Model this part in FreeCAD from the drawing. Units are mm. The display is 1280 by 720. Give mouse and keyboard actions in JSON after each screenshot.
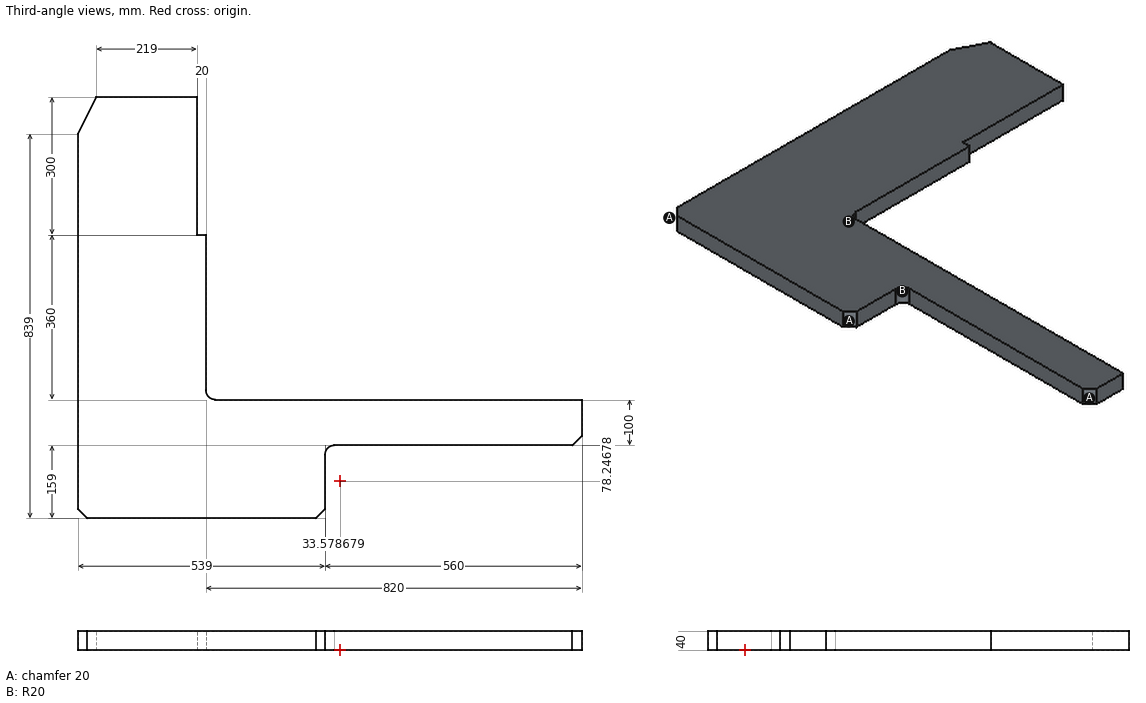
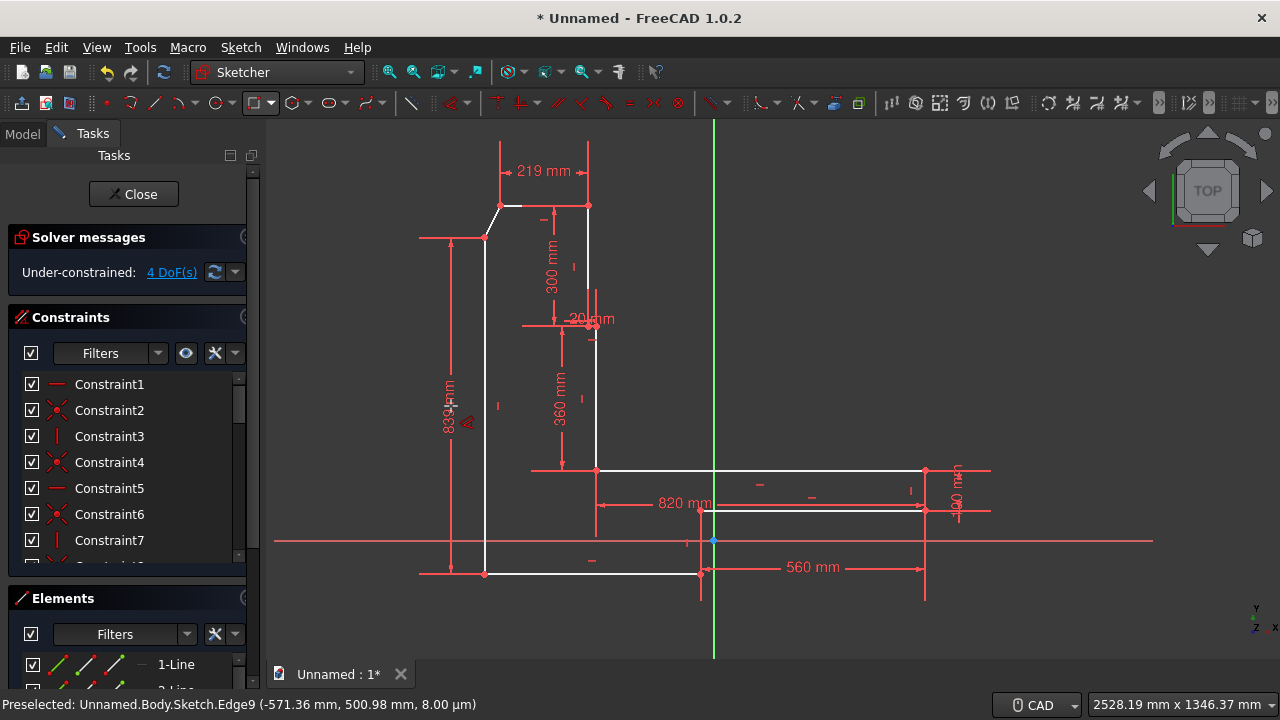
{"action": "left_click", "coordinate": [549, 574]}
{"action": "left_click", "coordinate": [593, 608]}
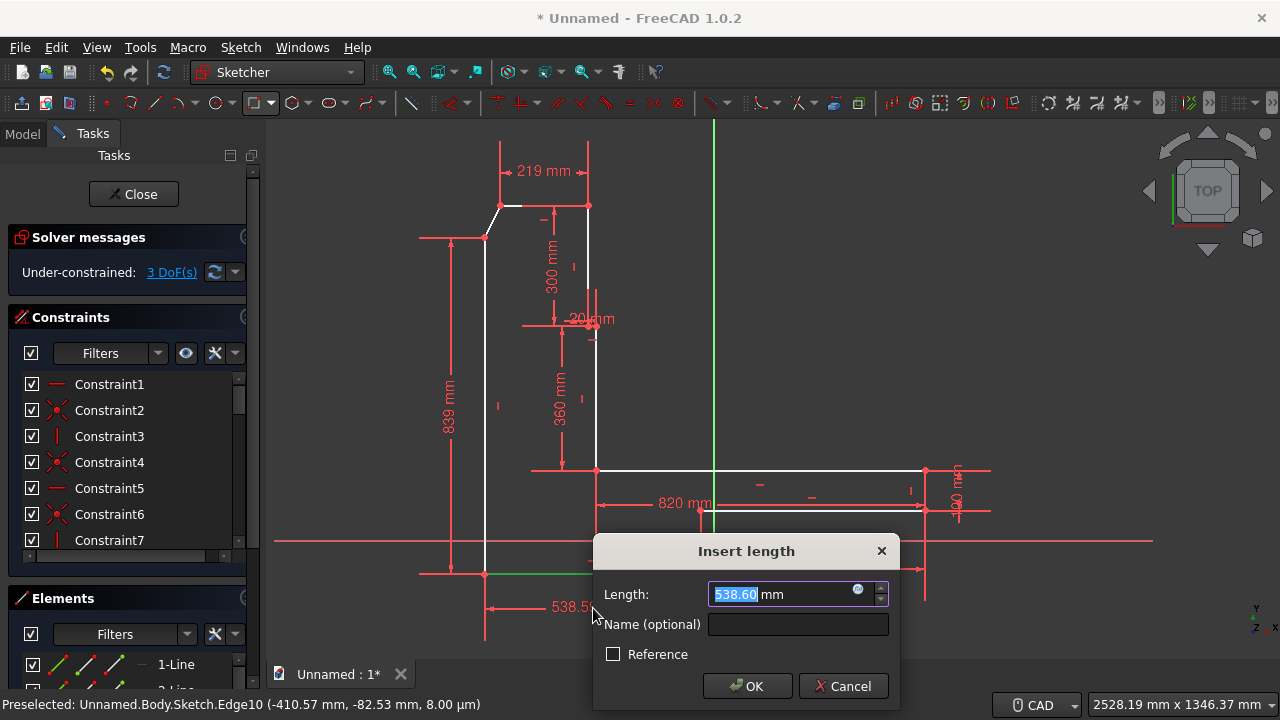
{"action": "type", "text": "539"}
{"action": "key", "text": "Return"}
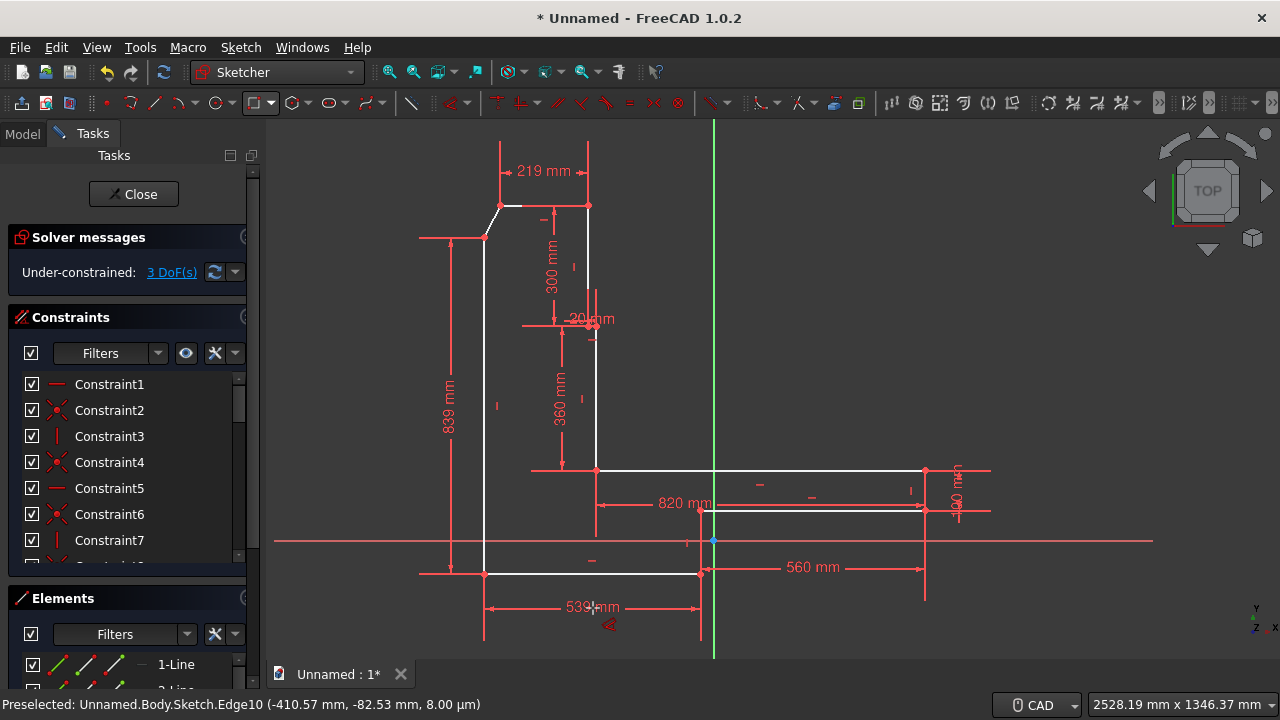
{"action": "left_click", "coordinate": [701, 555]}
{"action": "left_click", "coordinate": [667, 528]}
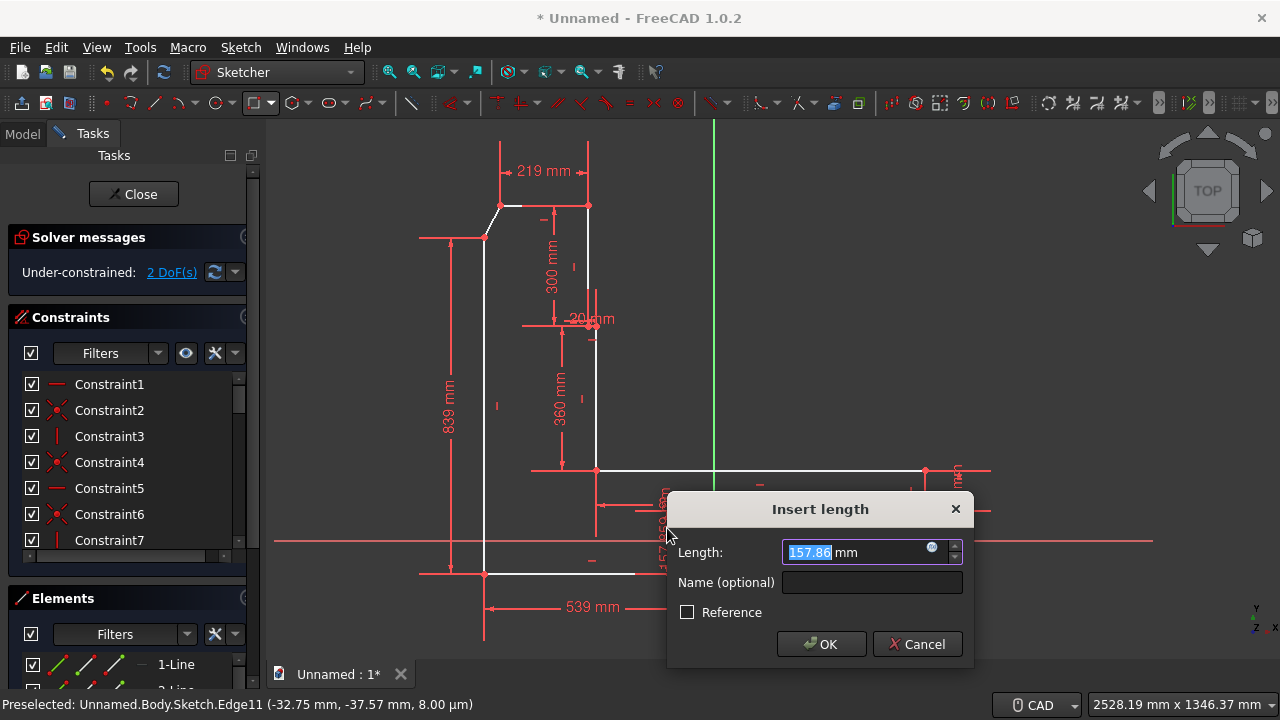
{"action": "type", "text": "159"}
{"action": "key", "text": "Return"}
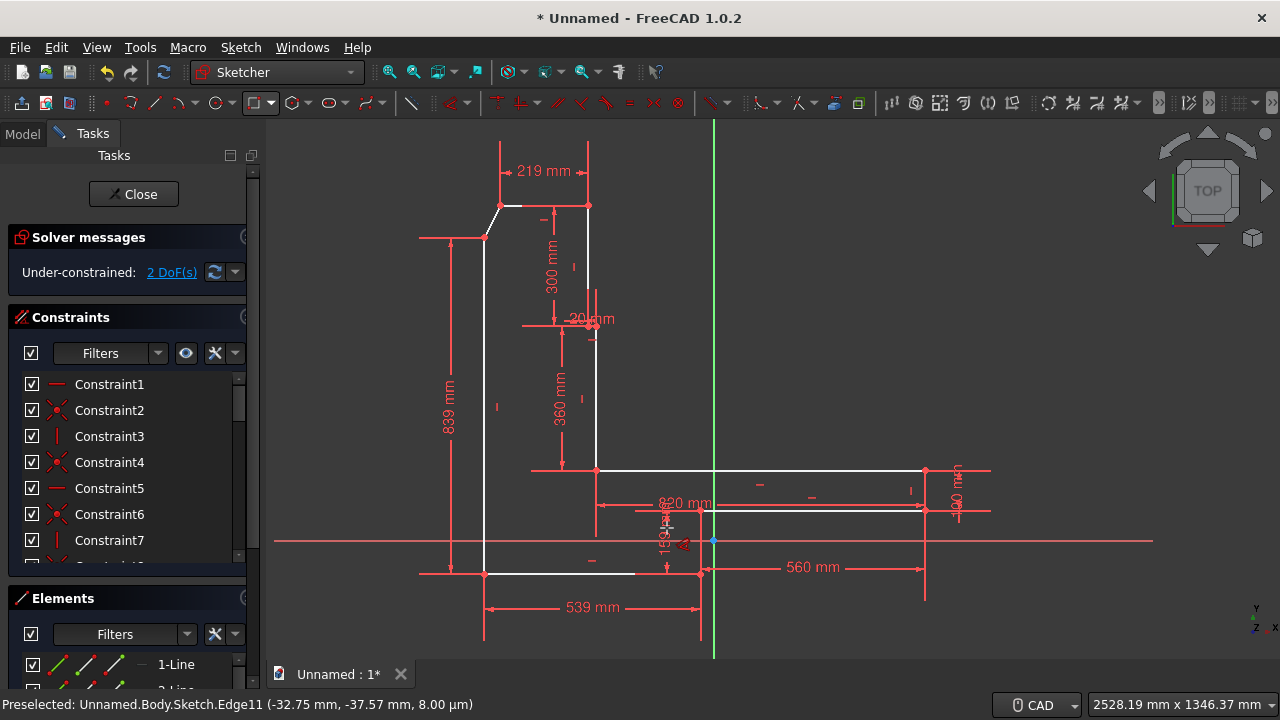
{"action": "scroll", "coordinate": [701, 511], "scroll_direction": "up", "scroll_amount": 2}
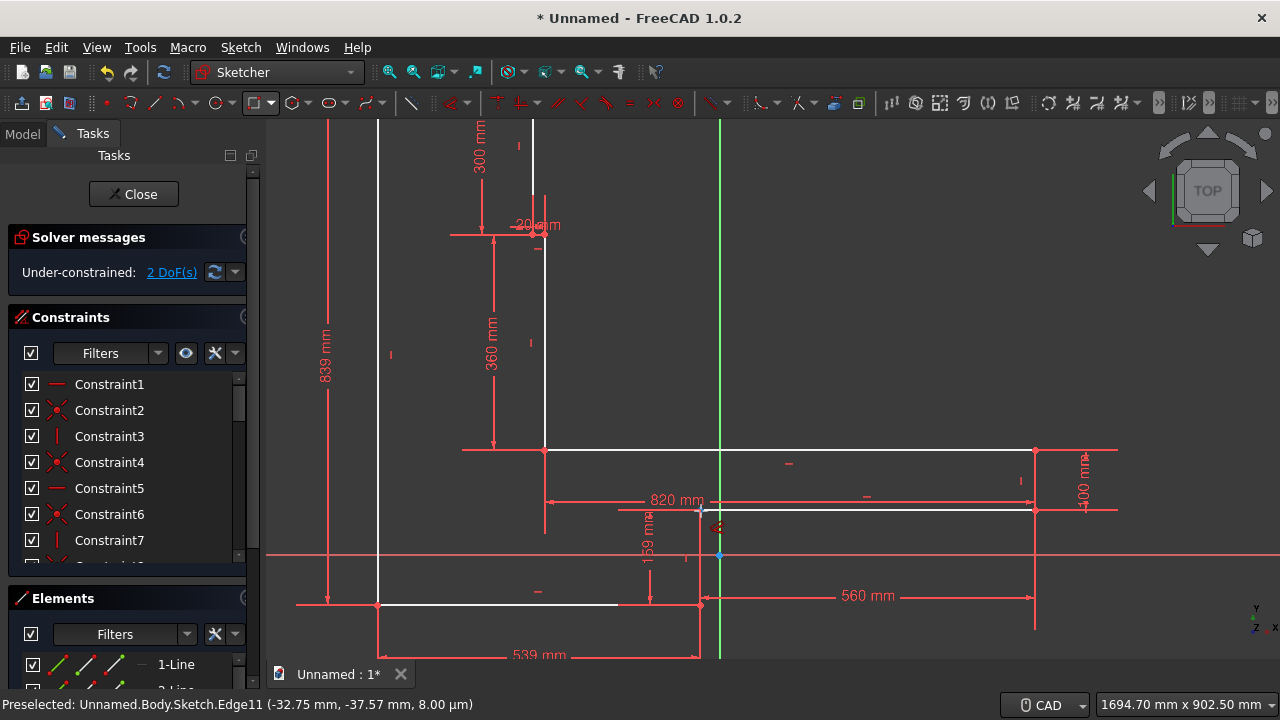
{"action": "left_click", "coordinate": [700, 510]}
{"action": "left_click", "coordinate": [754, 533]}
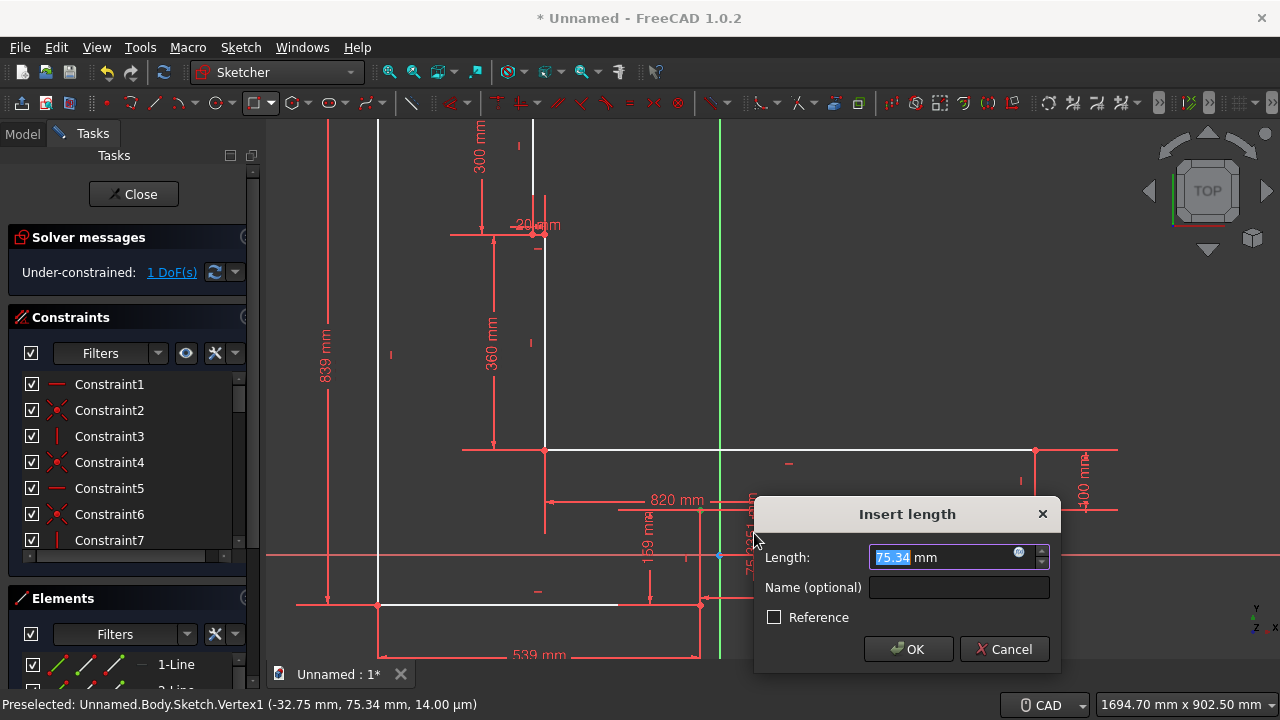
{"action": "type", "text": "78.24678"}
{"action": "key", "text": "Return"}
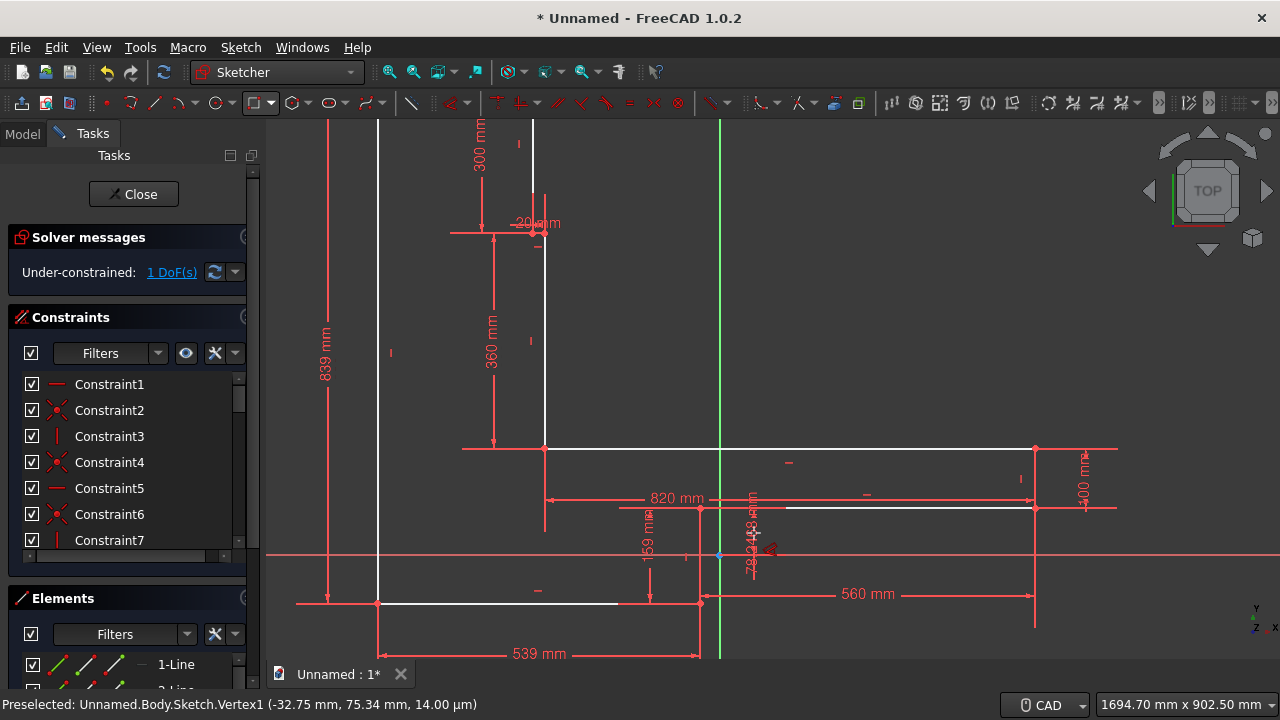
{"action": "scroll", "coordinate": [700, 508], "scroll_direction": "up", "scroll_amount": 4}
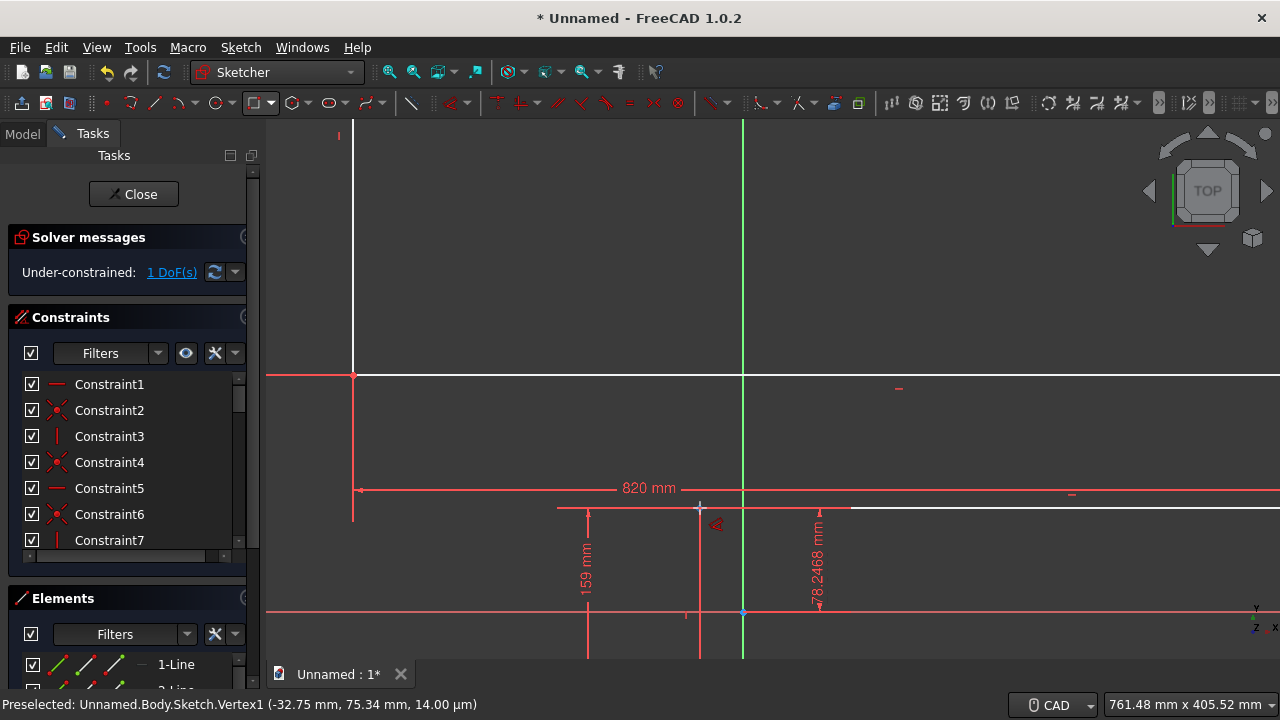
{"action": "left_click", "coordinate": [700, 508]}
{"action": "left_click", "coordinate": [721, 474]}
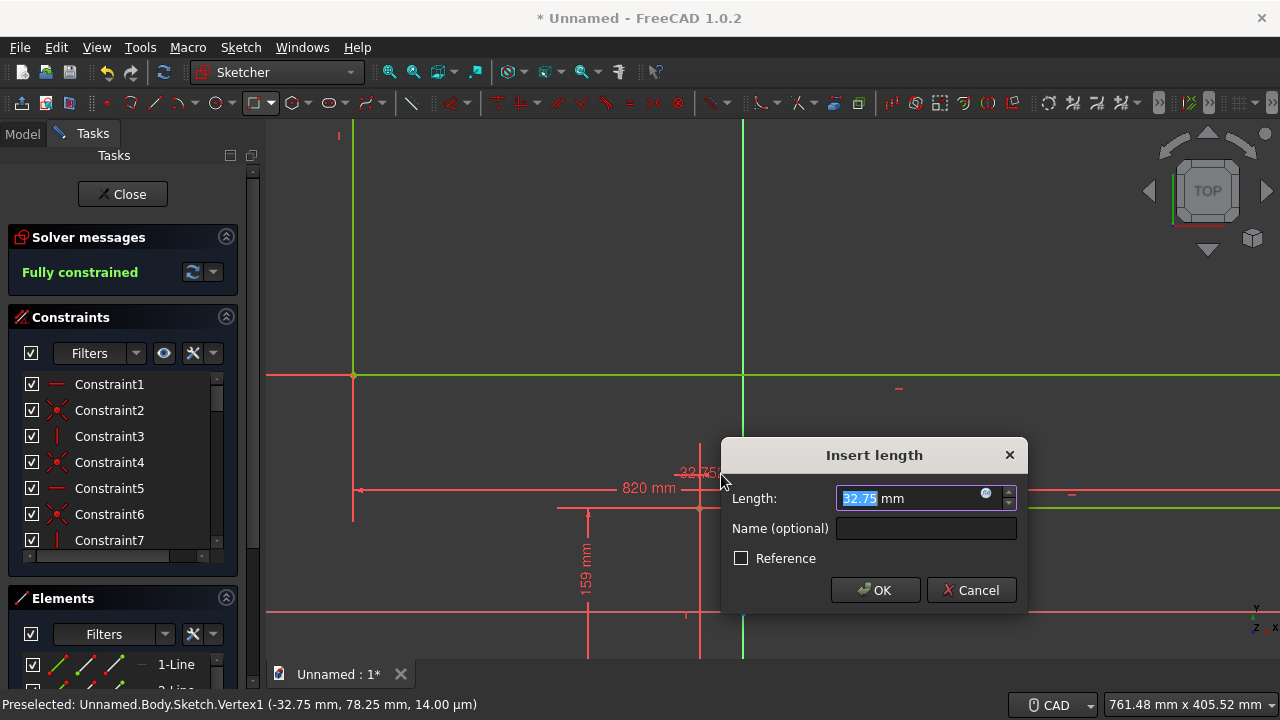
{"action": "type", "text": "33.578679"}
{"action": "key", "text": "Return"}
{"action": "key", "text": "Escape"}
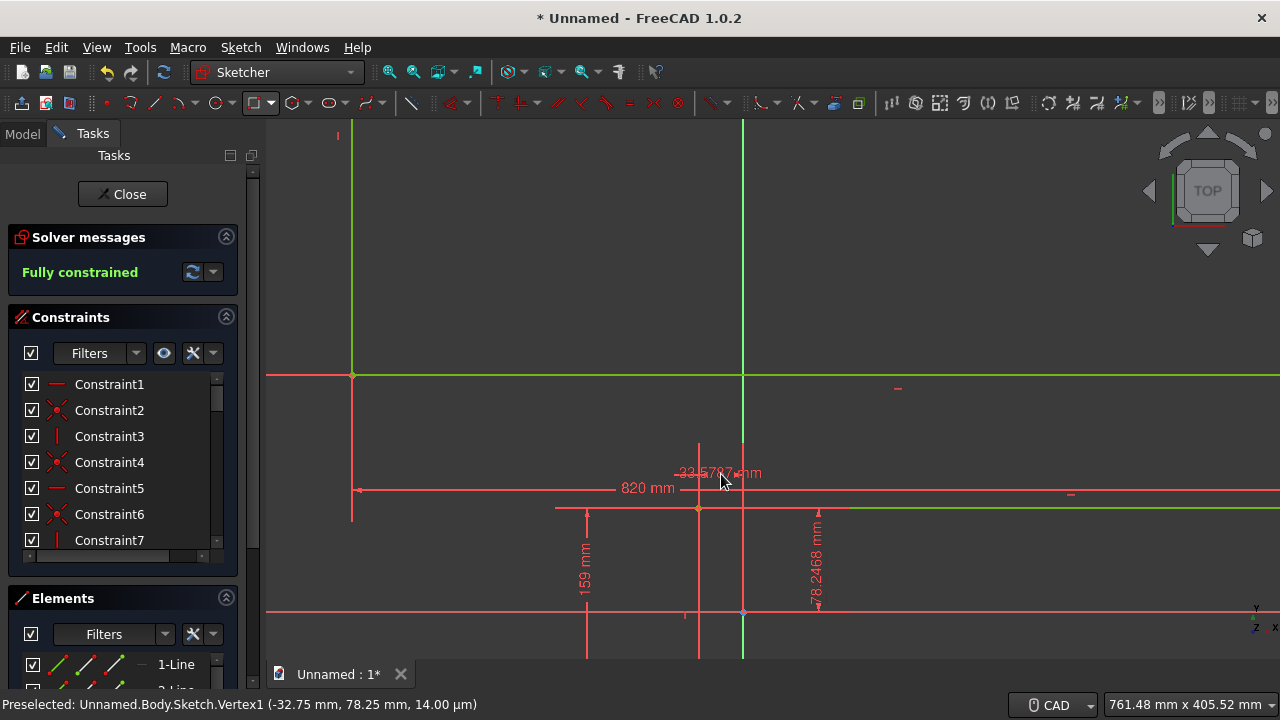
{"action": "left_click", "coordinate": [123, 194]}